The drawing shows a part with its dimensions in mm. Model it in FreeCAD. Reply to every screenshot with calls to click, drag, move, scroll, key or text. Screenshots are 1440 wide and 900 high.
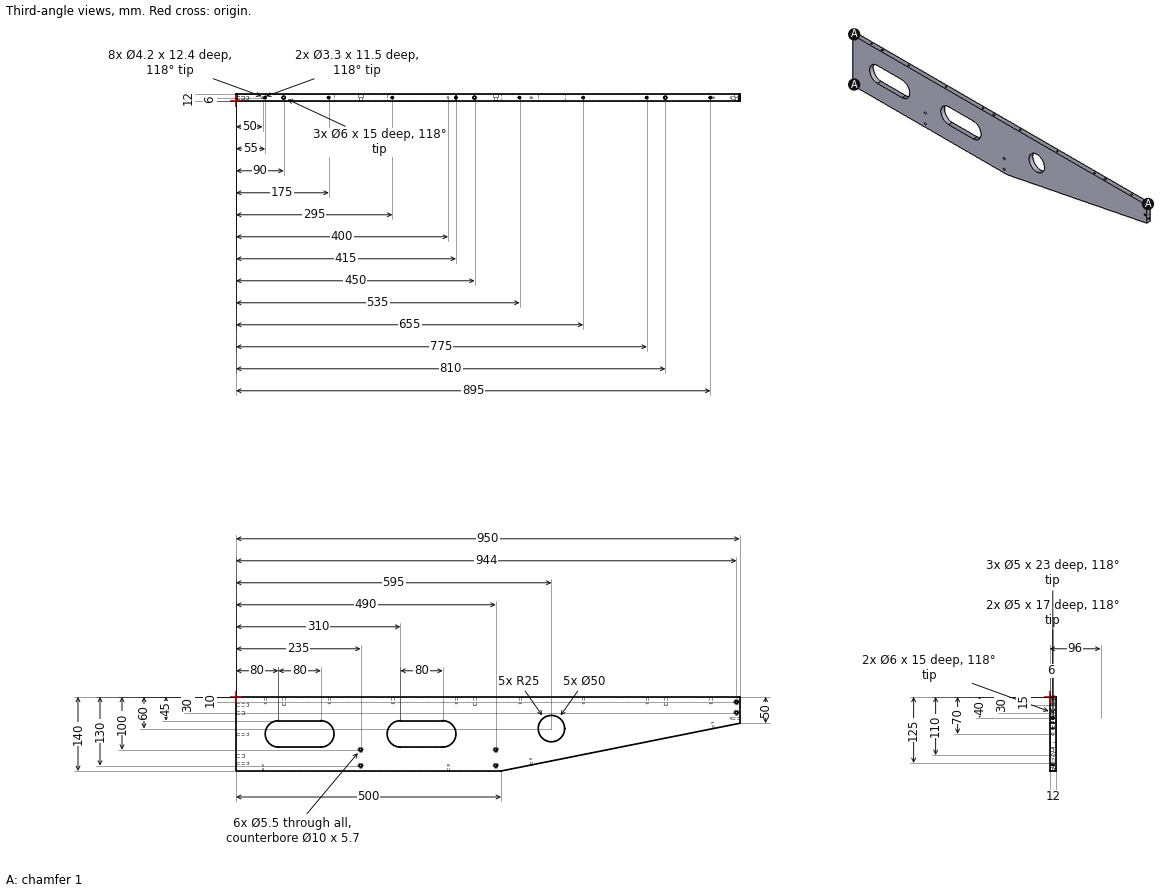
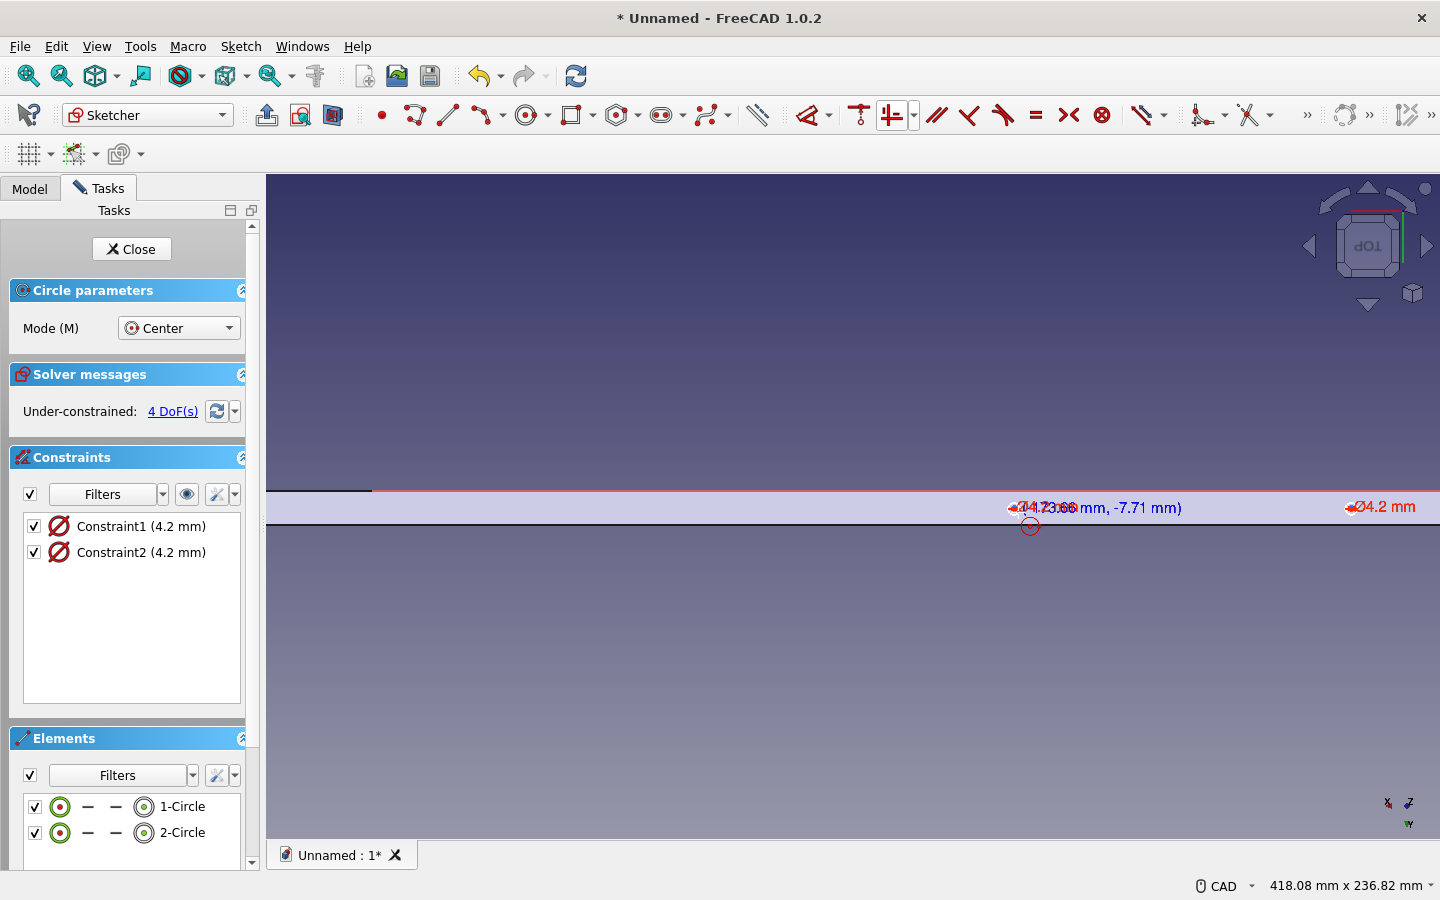
scroll(677, 508, up, 7)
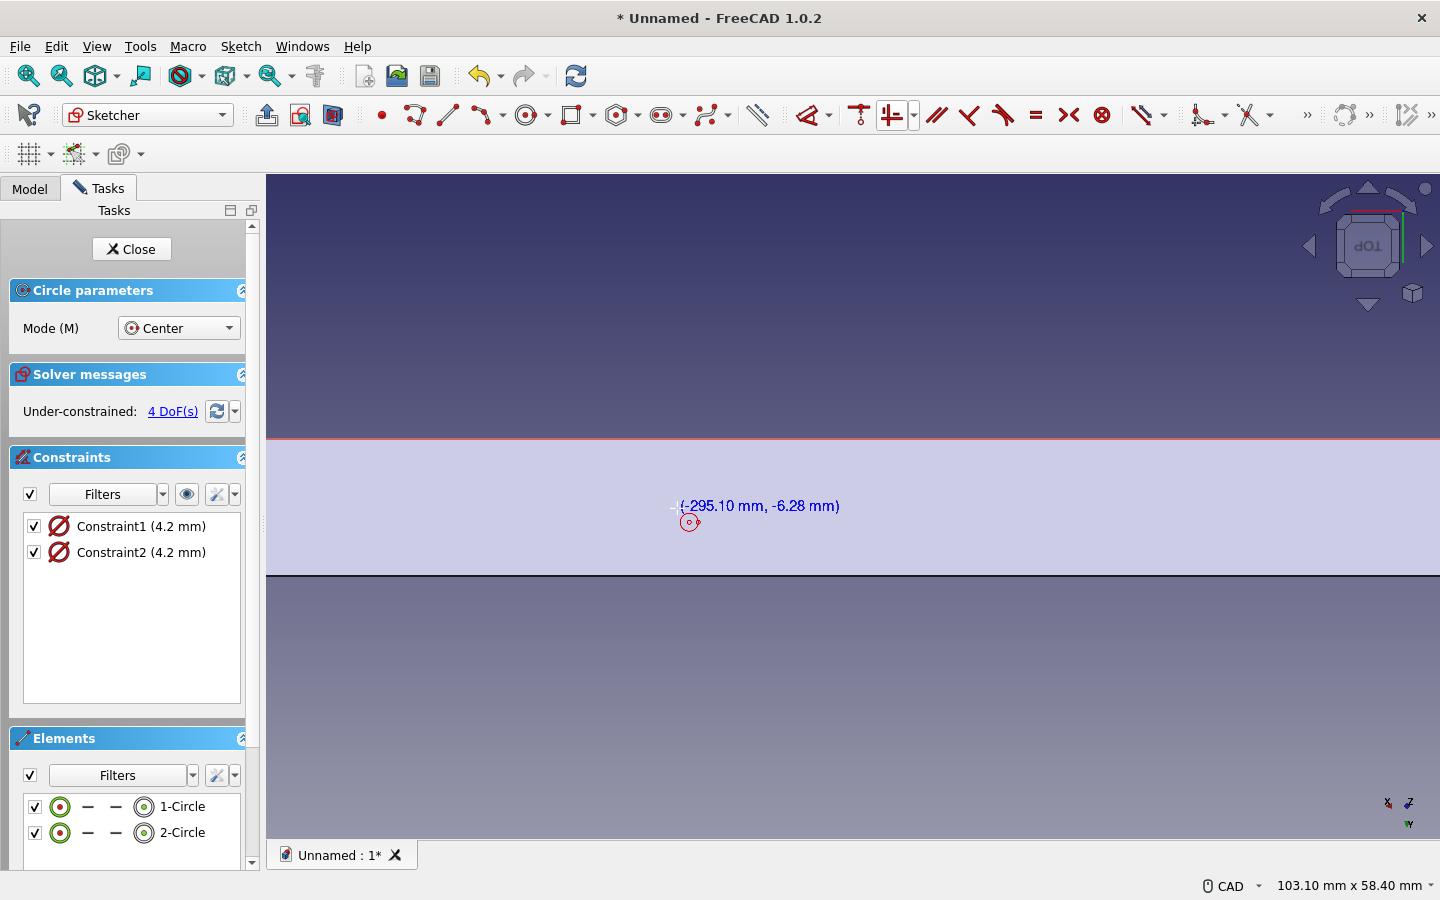
scroll(933, 508, down, 13)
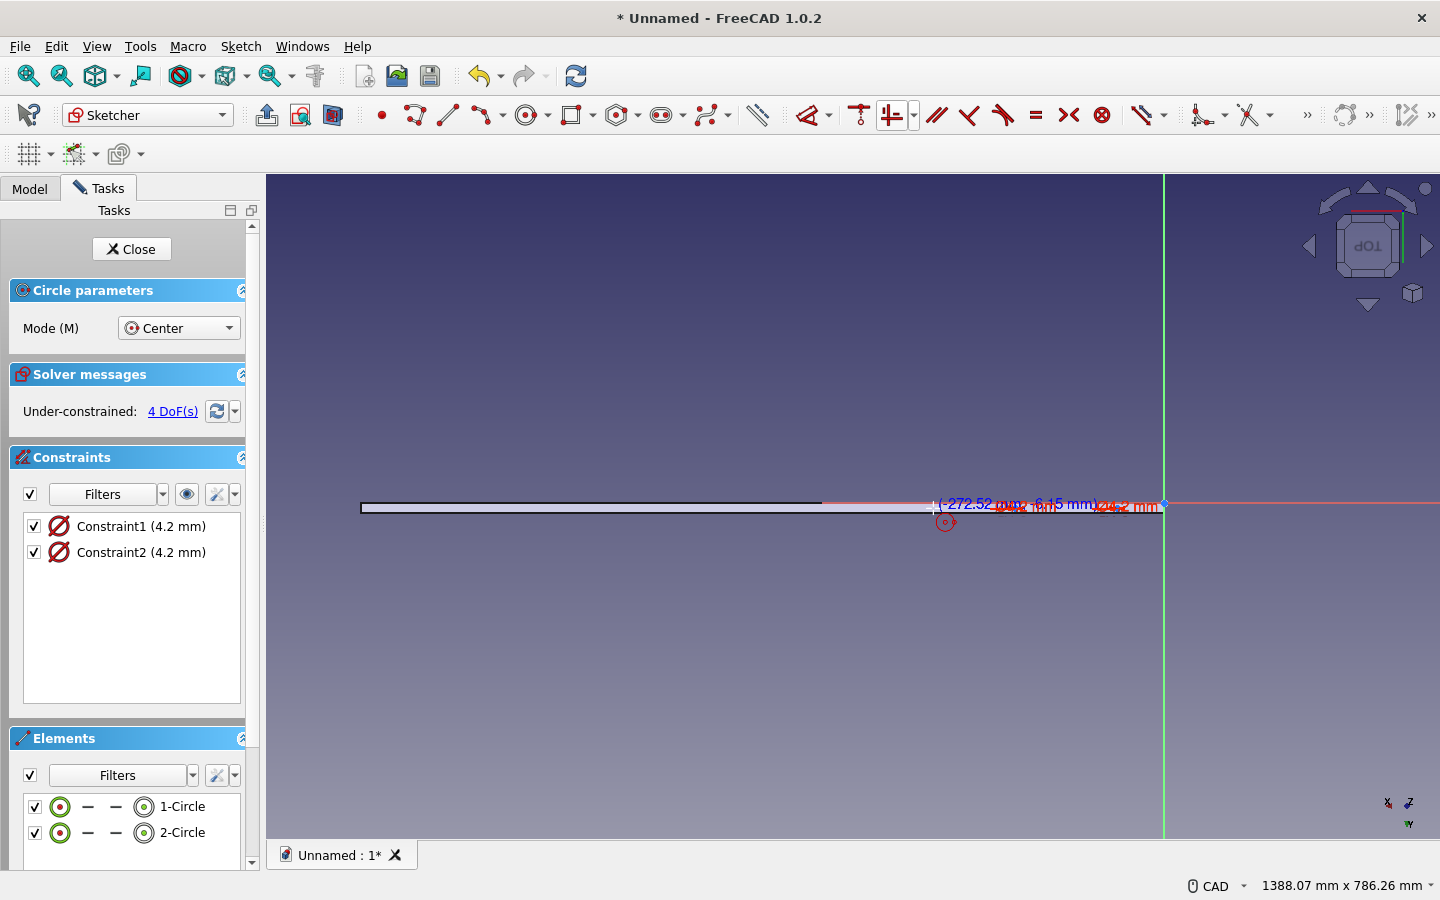
scroll(915, 508, up, 6)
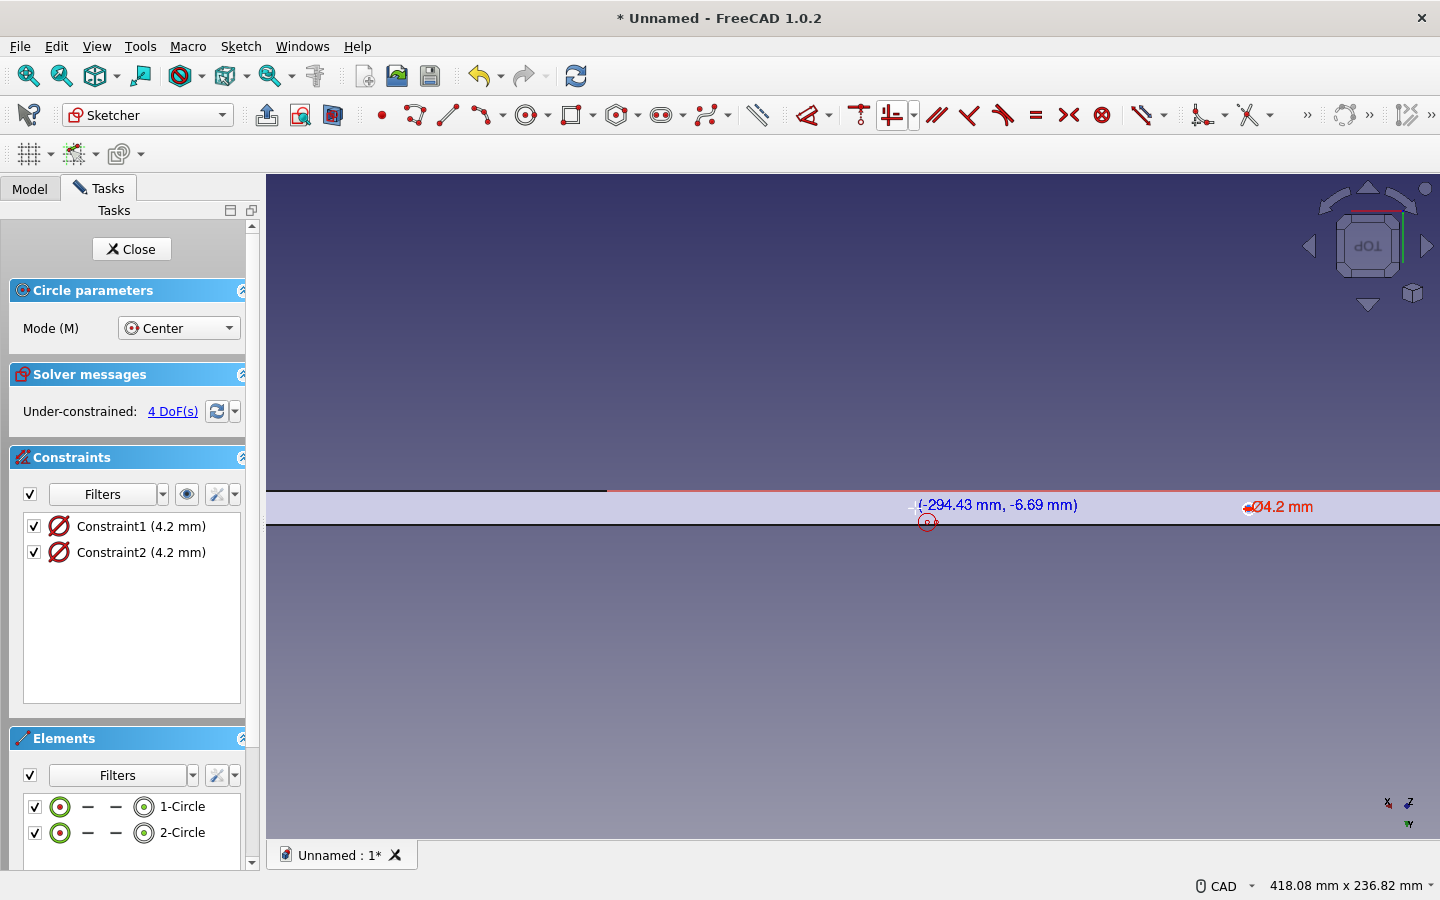
click(912, 508)
move(916, 512)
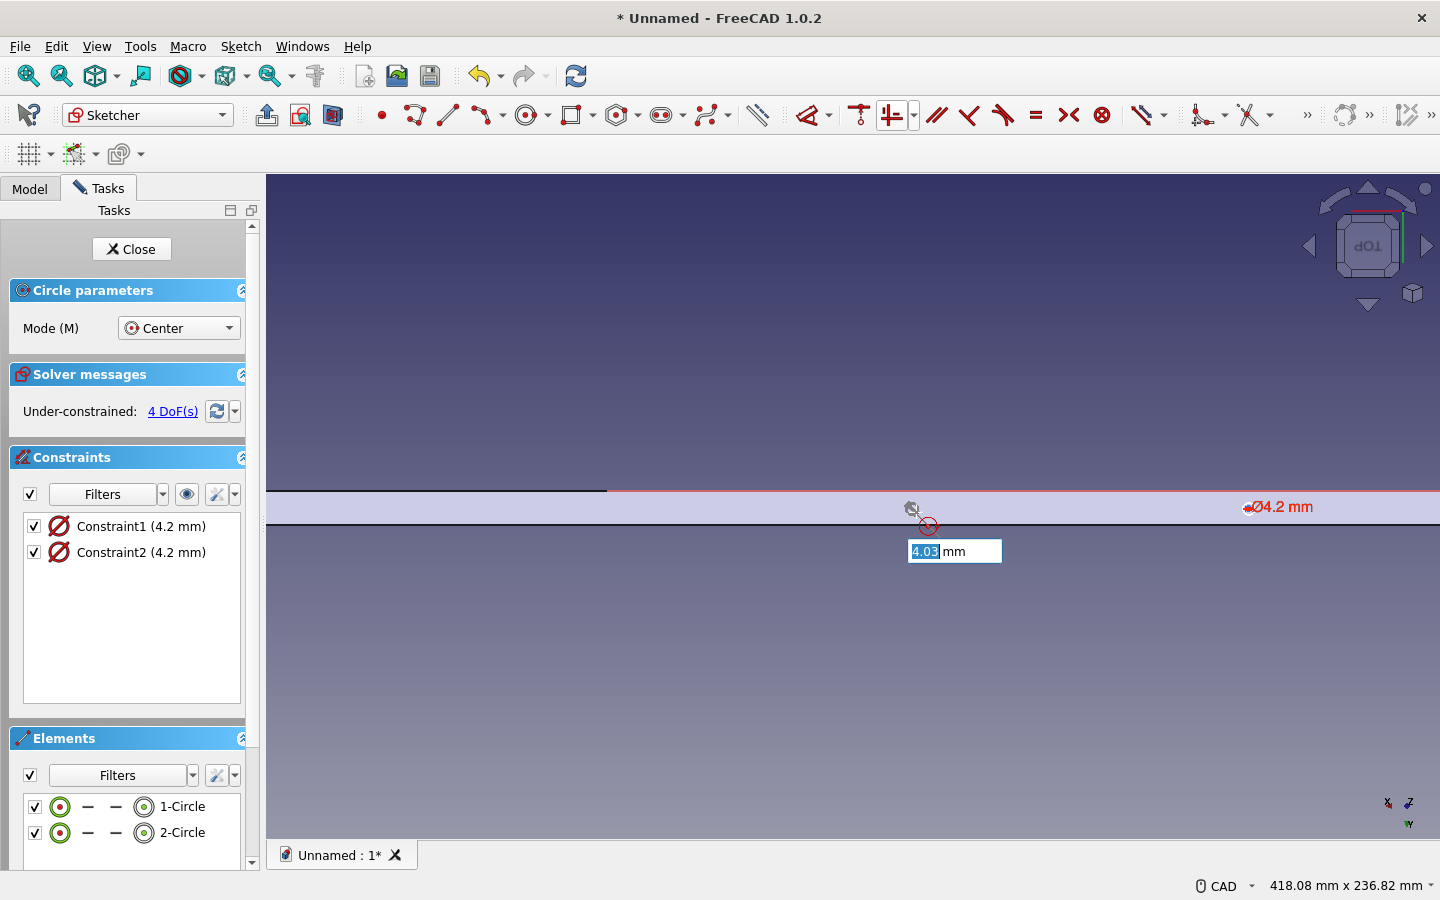
text(4.2)
key(Return)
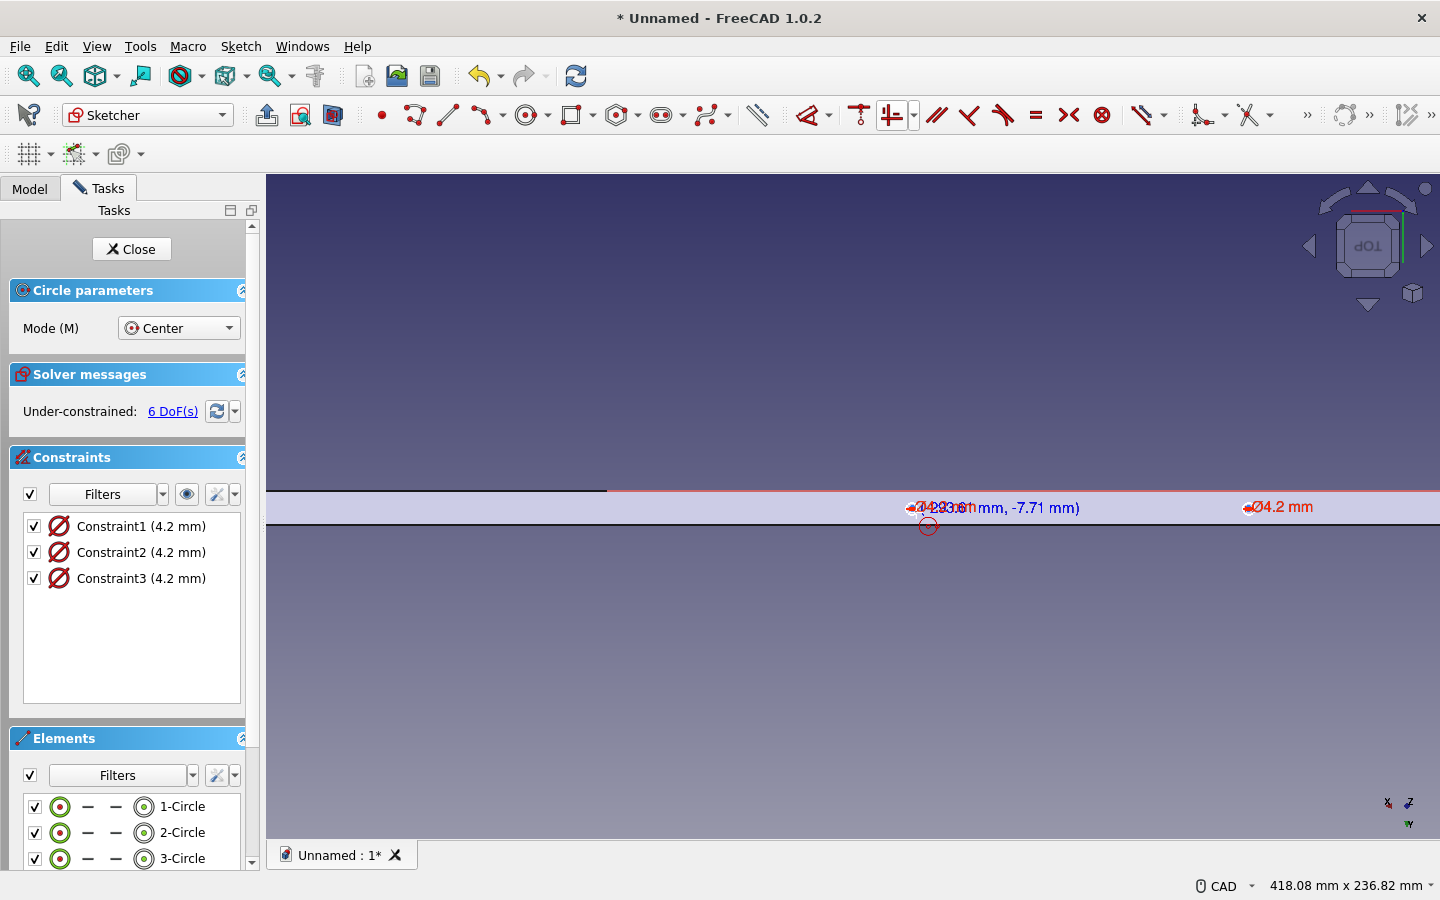
scroll(575, 508, up, 7)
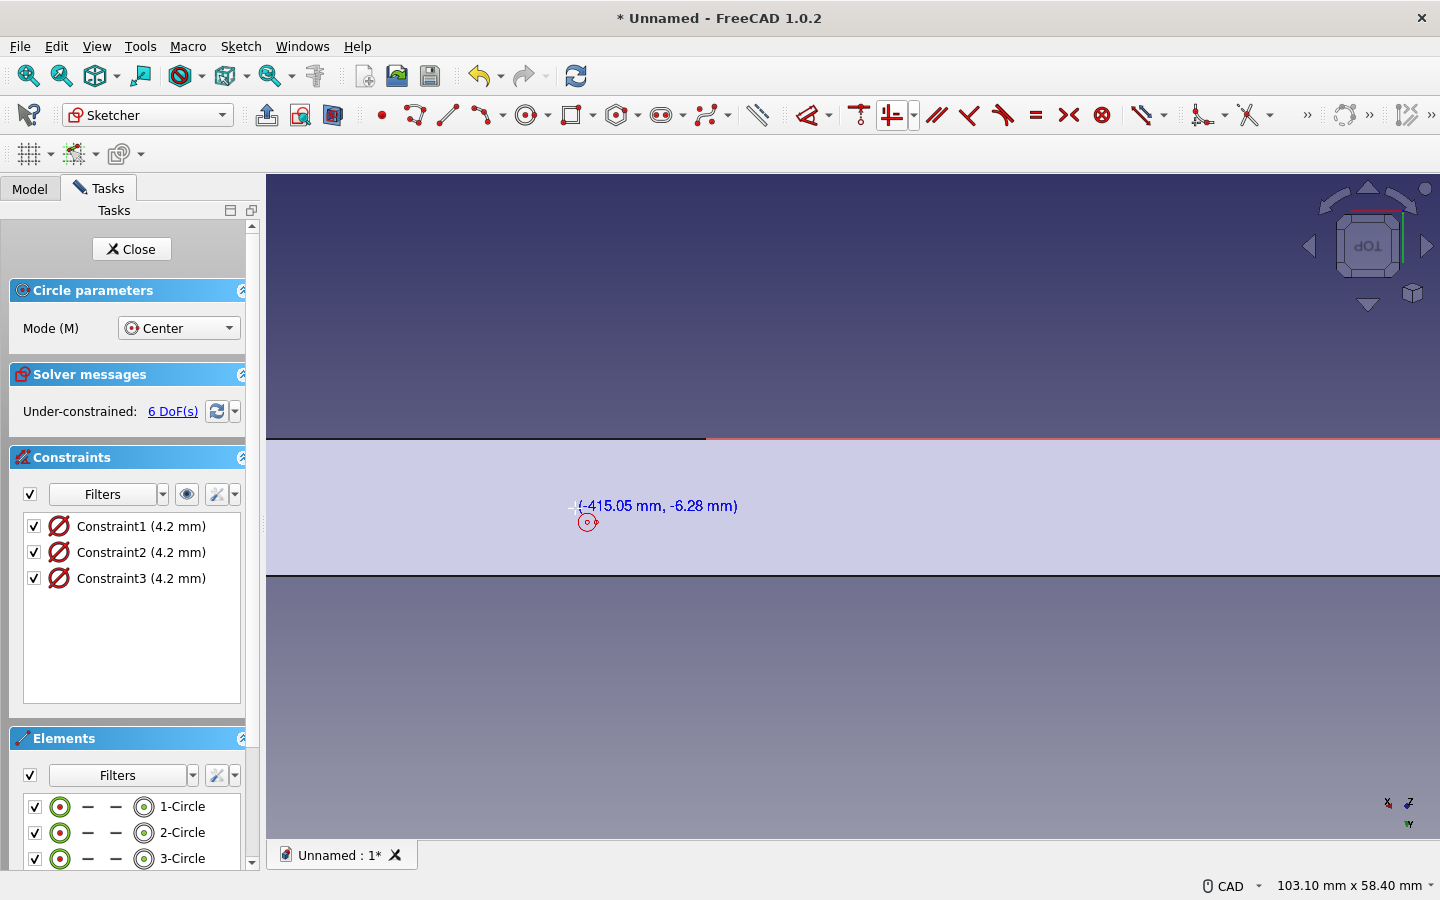
scroll(832, 508, down, 13)